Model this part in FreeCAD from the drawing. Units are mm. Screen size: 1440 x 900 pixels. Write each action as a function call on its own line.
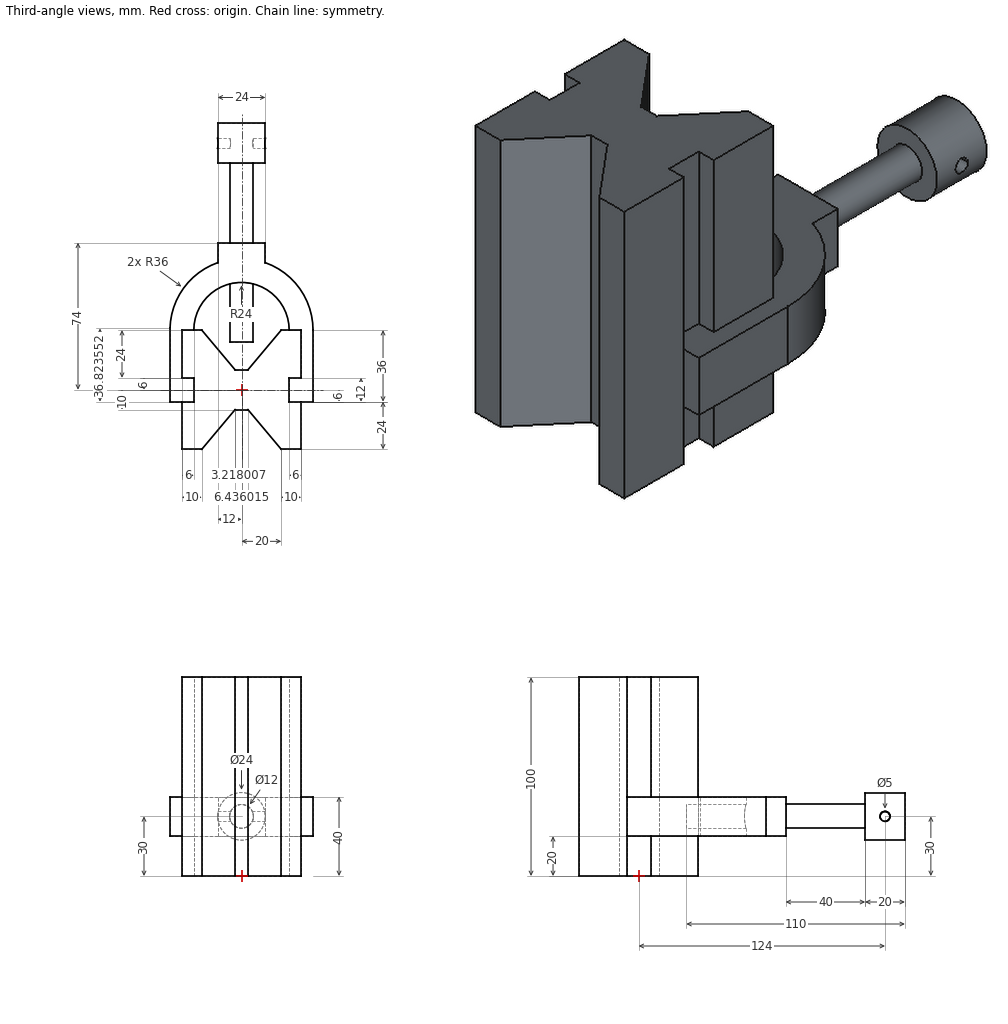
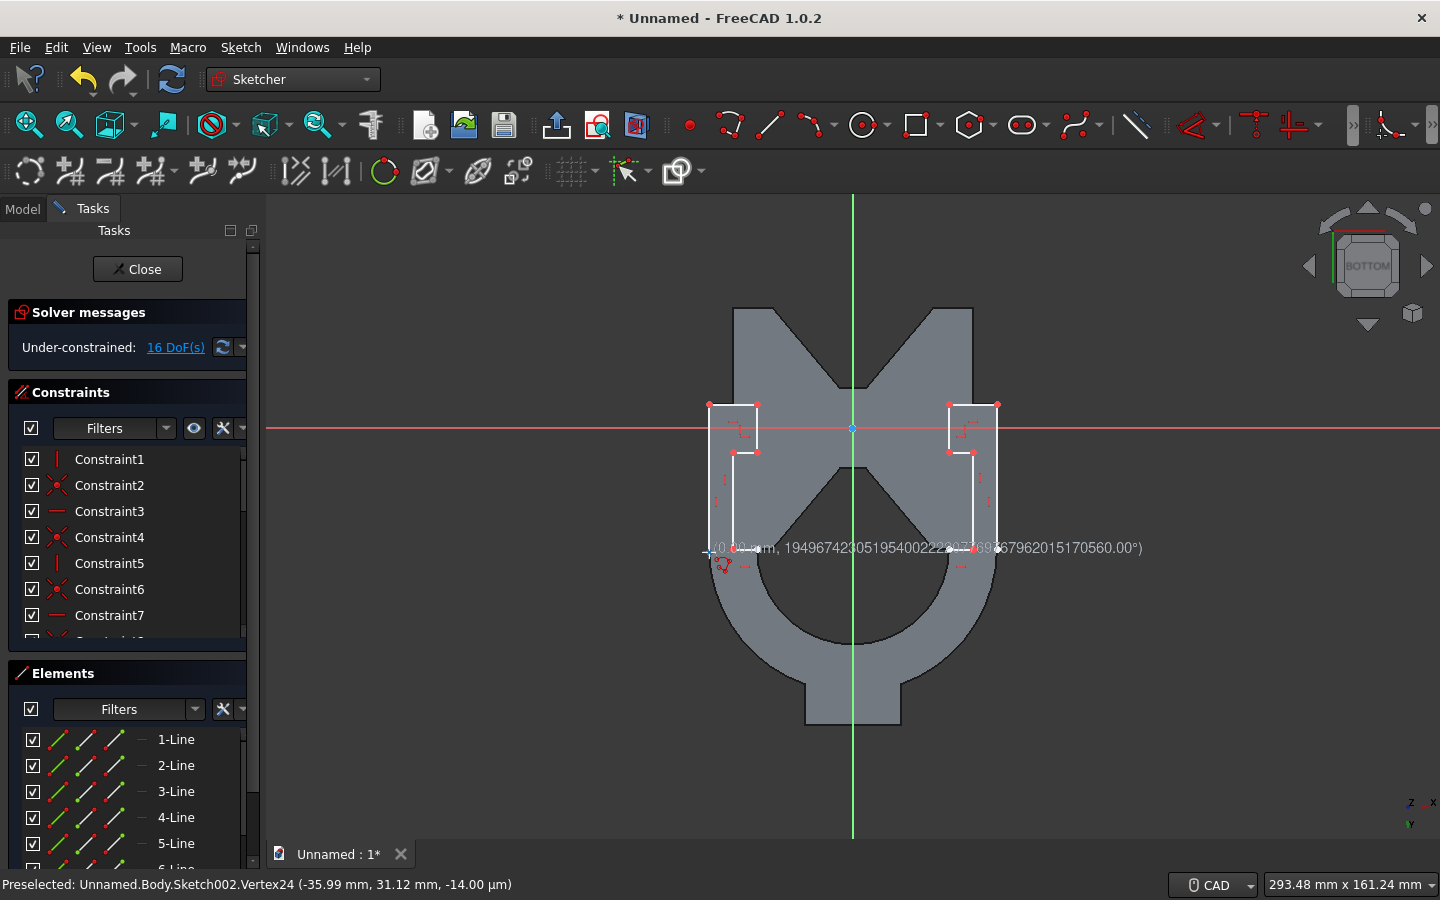
click(805, 684)
click(805, 725)
click(901, 725)
click(901, 684)
right_click(901, 684)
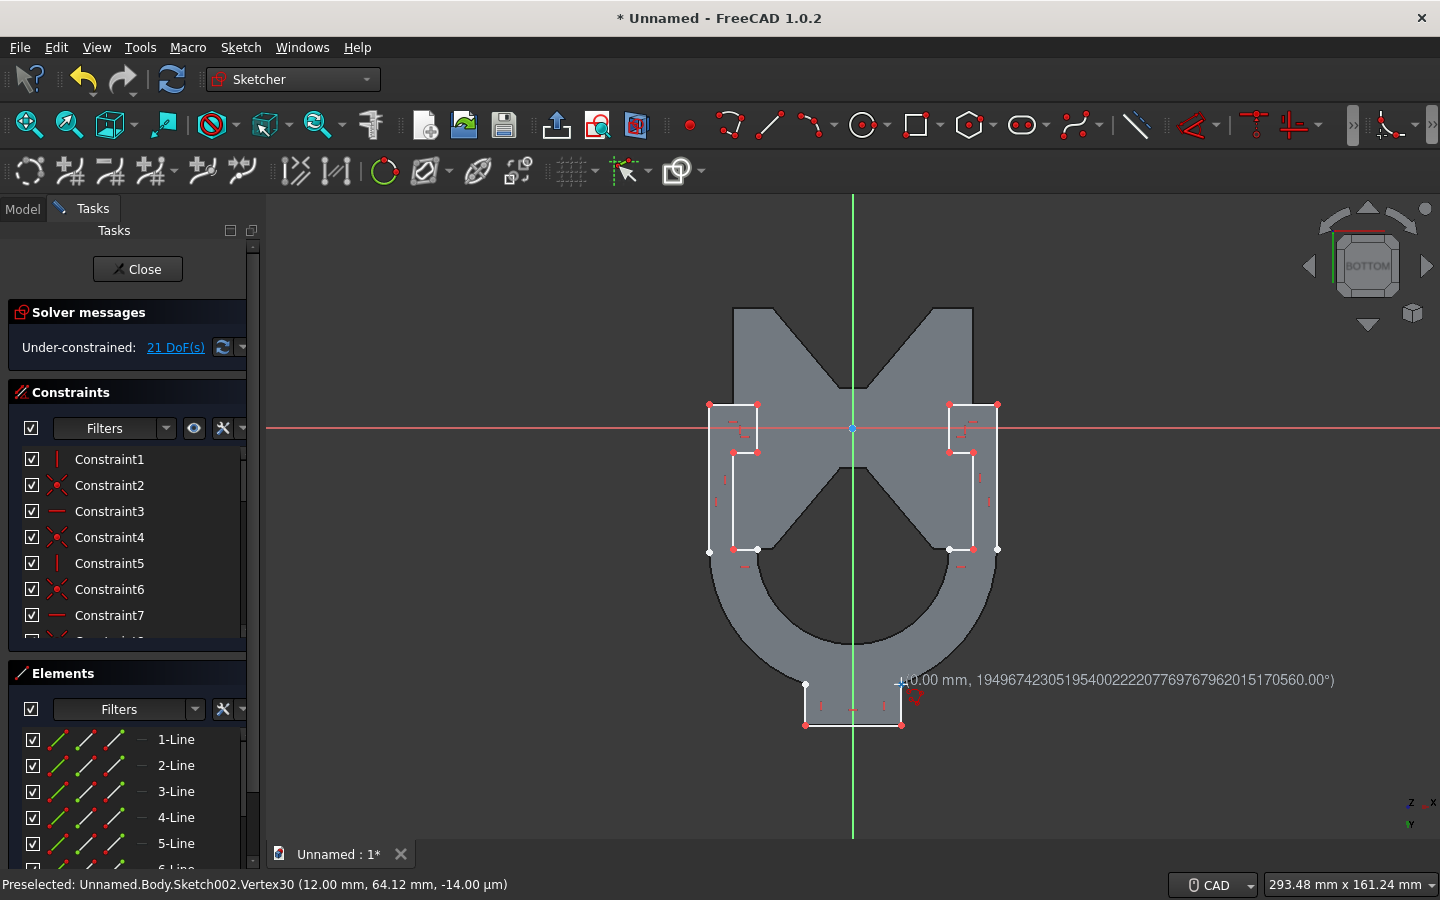
click(810, 126)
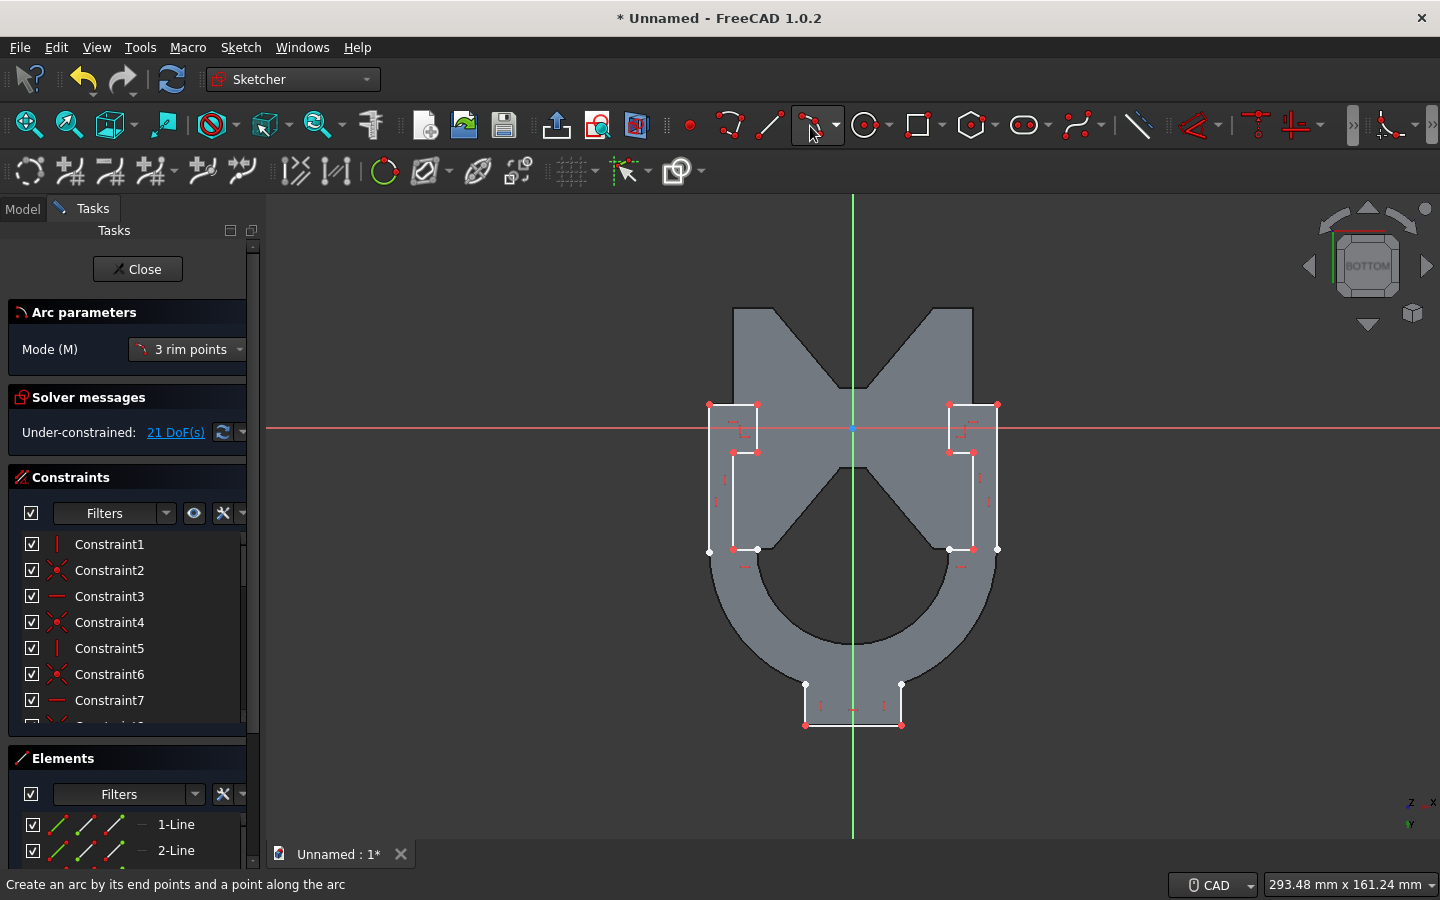
scroll(949, 549, up, 2)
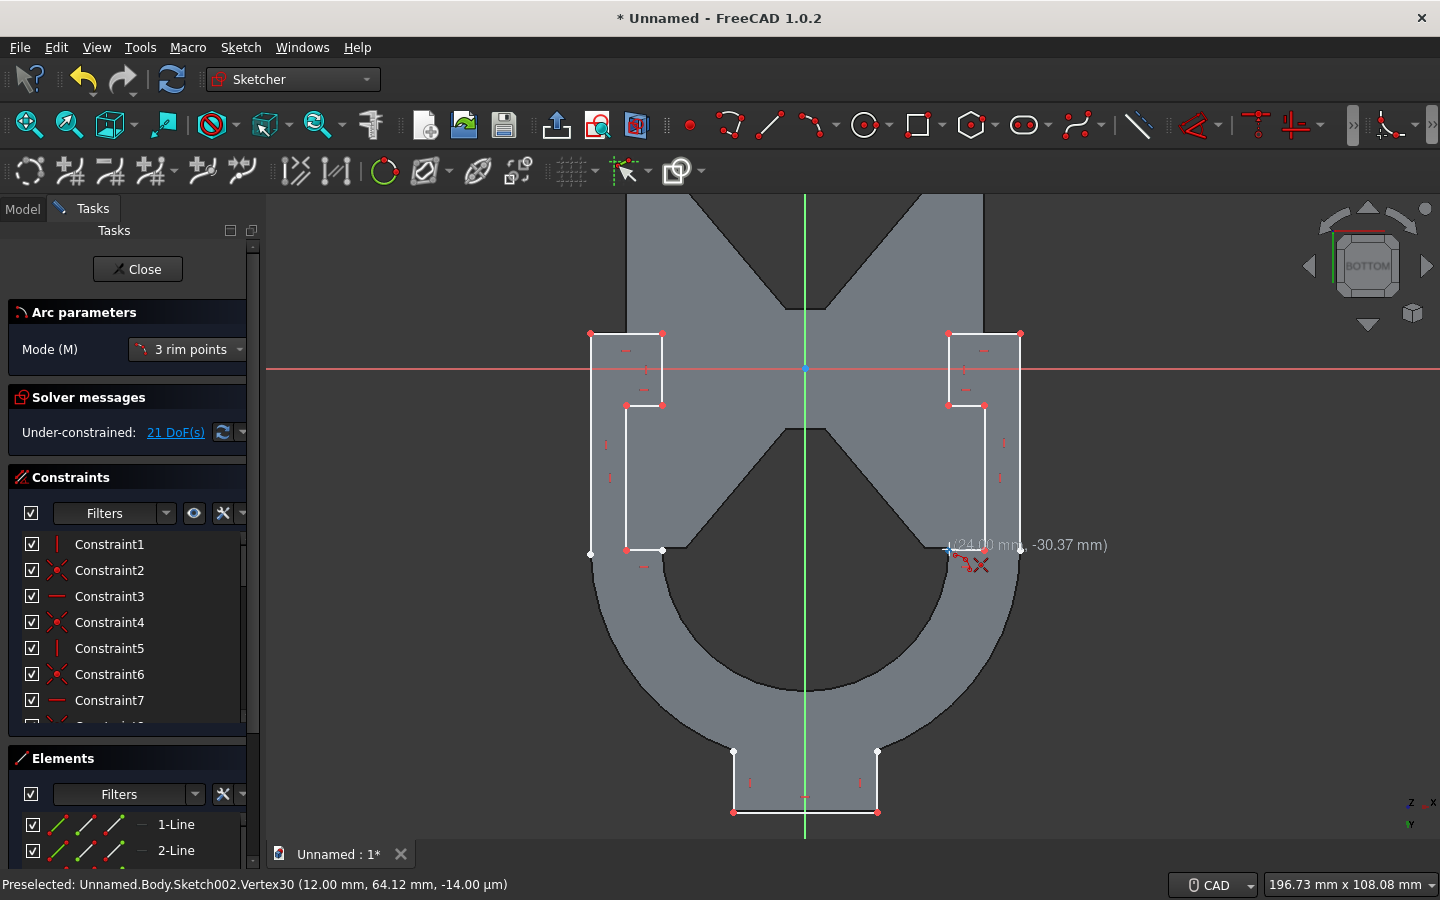
click(949, 550)
click(662, 550)
click(761, 684)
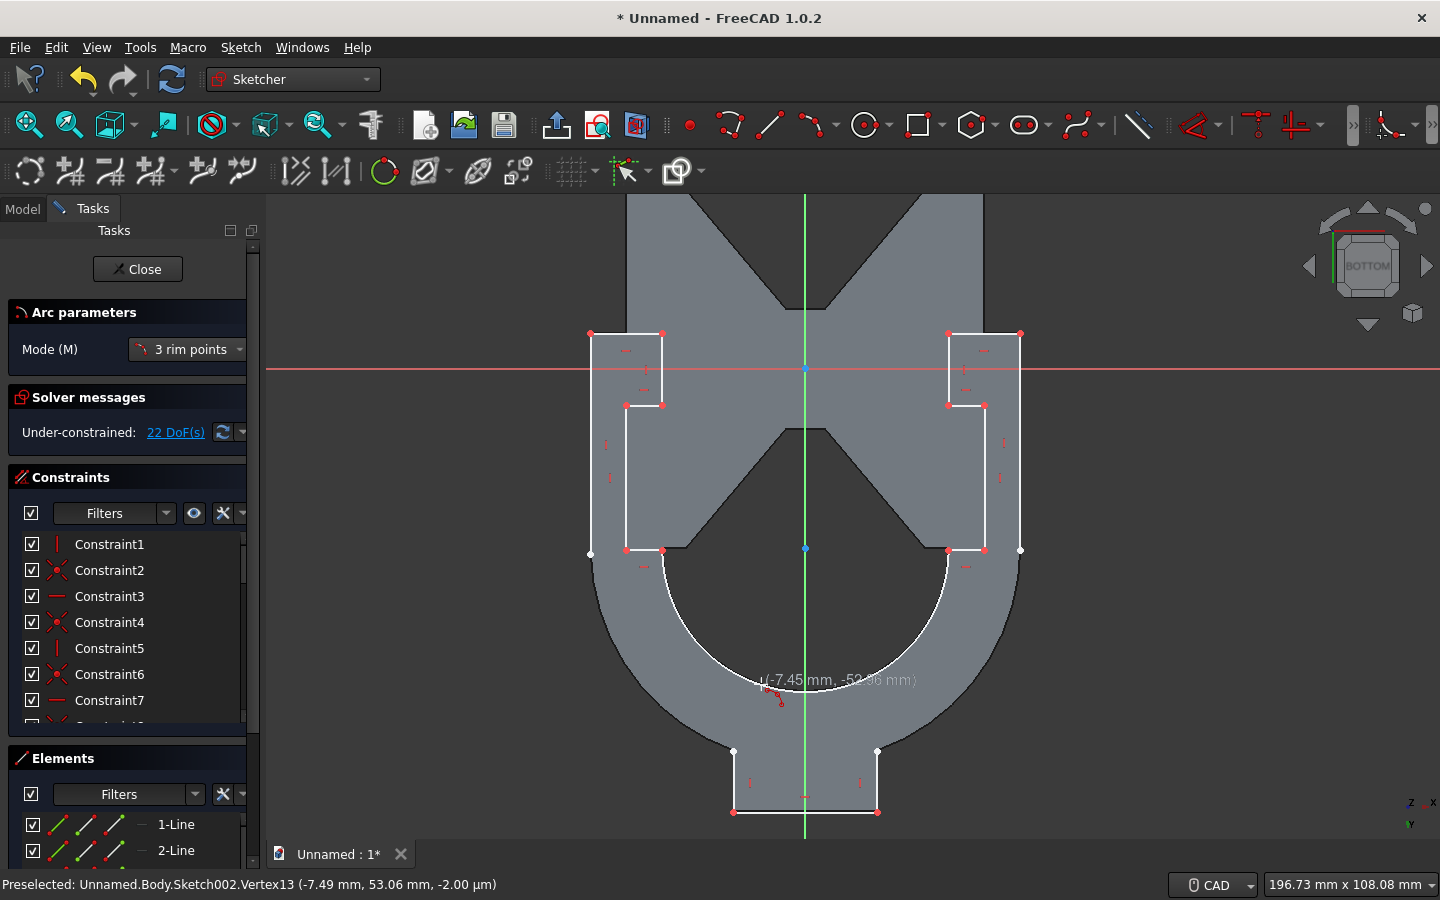
click(591, 555)
click(734, 752)
click(631, 674)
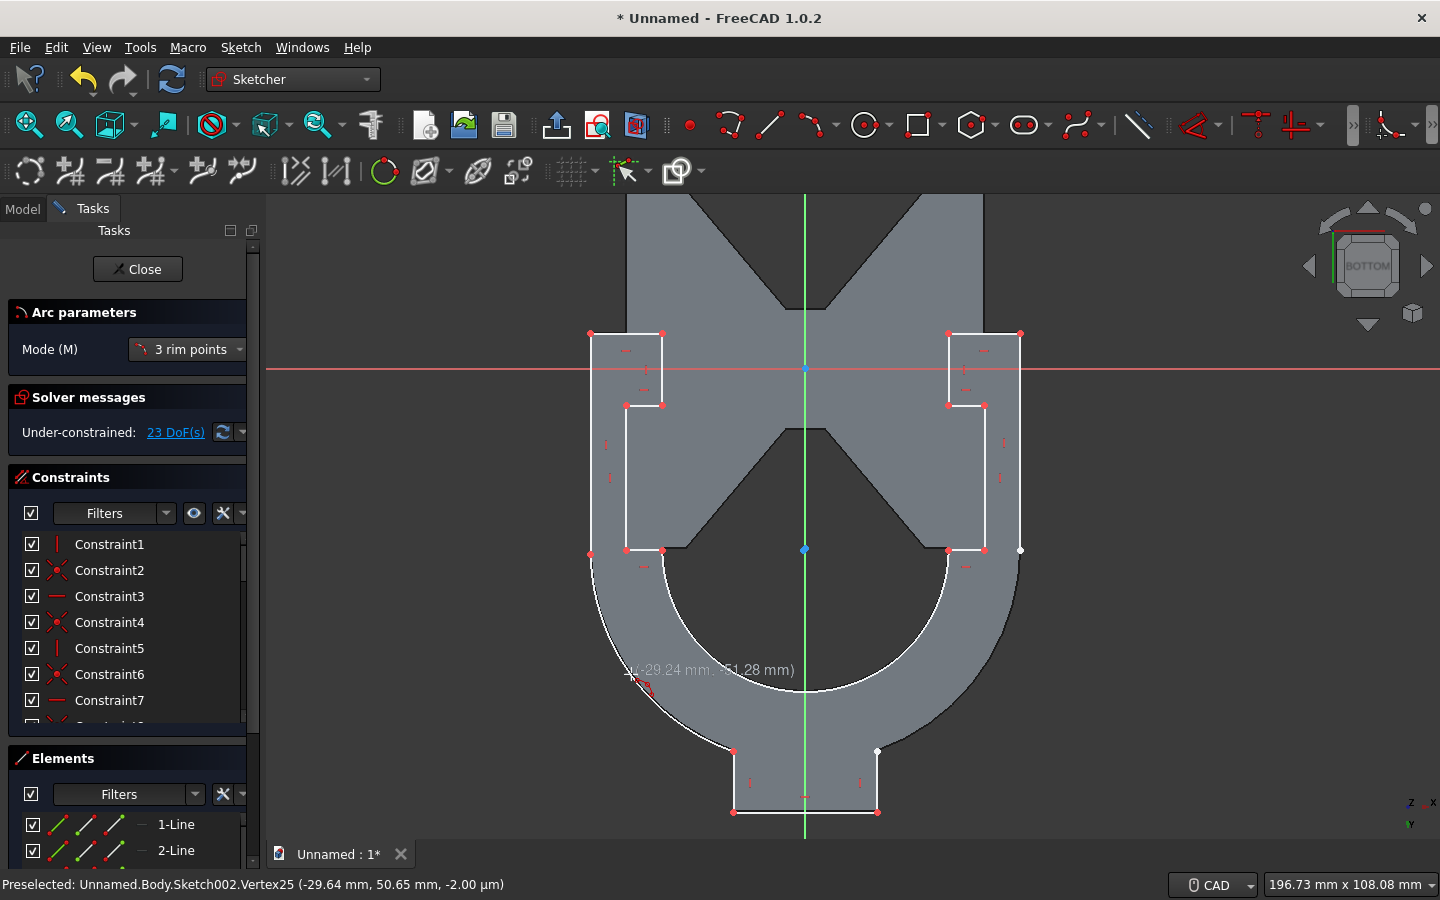
click(877, 752)
click(1020, 550)
click(981, 672)
key(Escape)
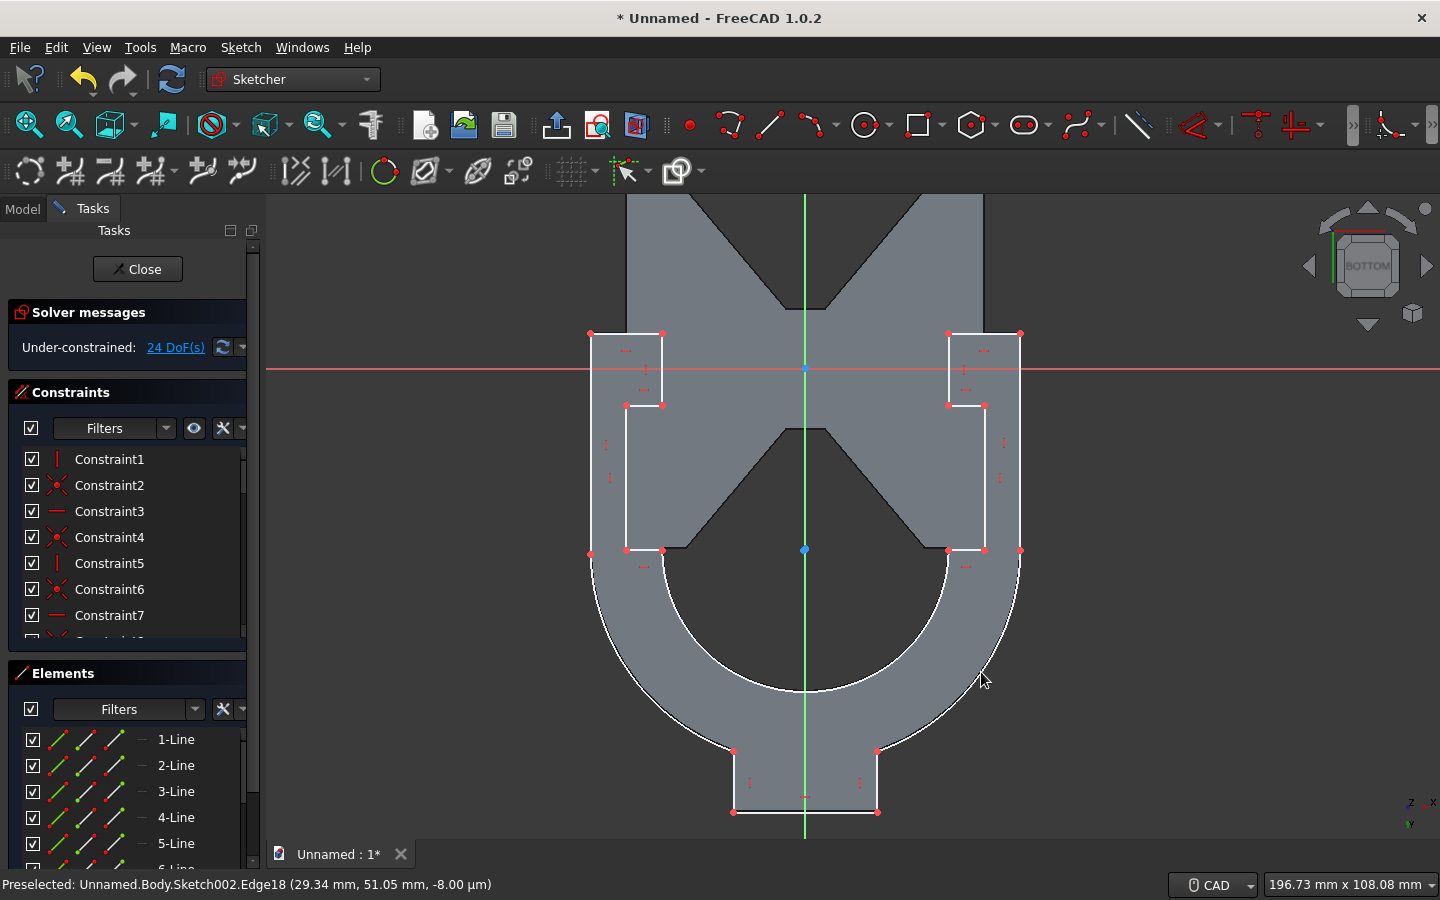
click(1020, 485)